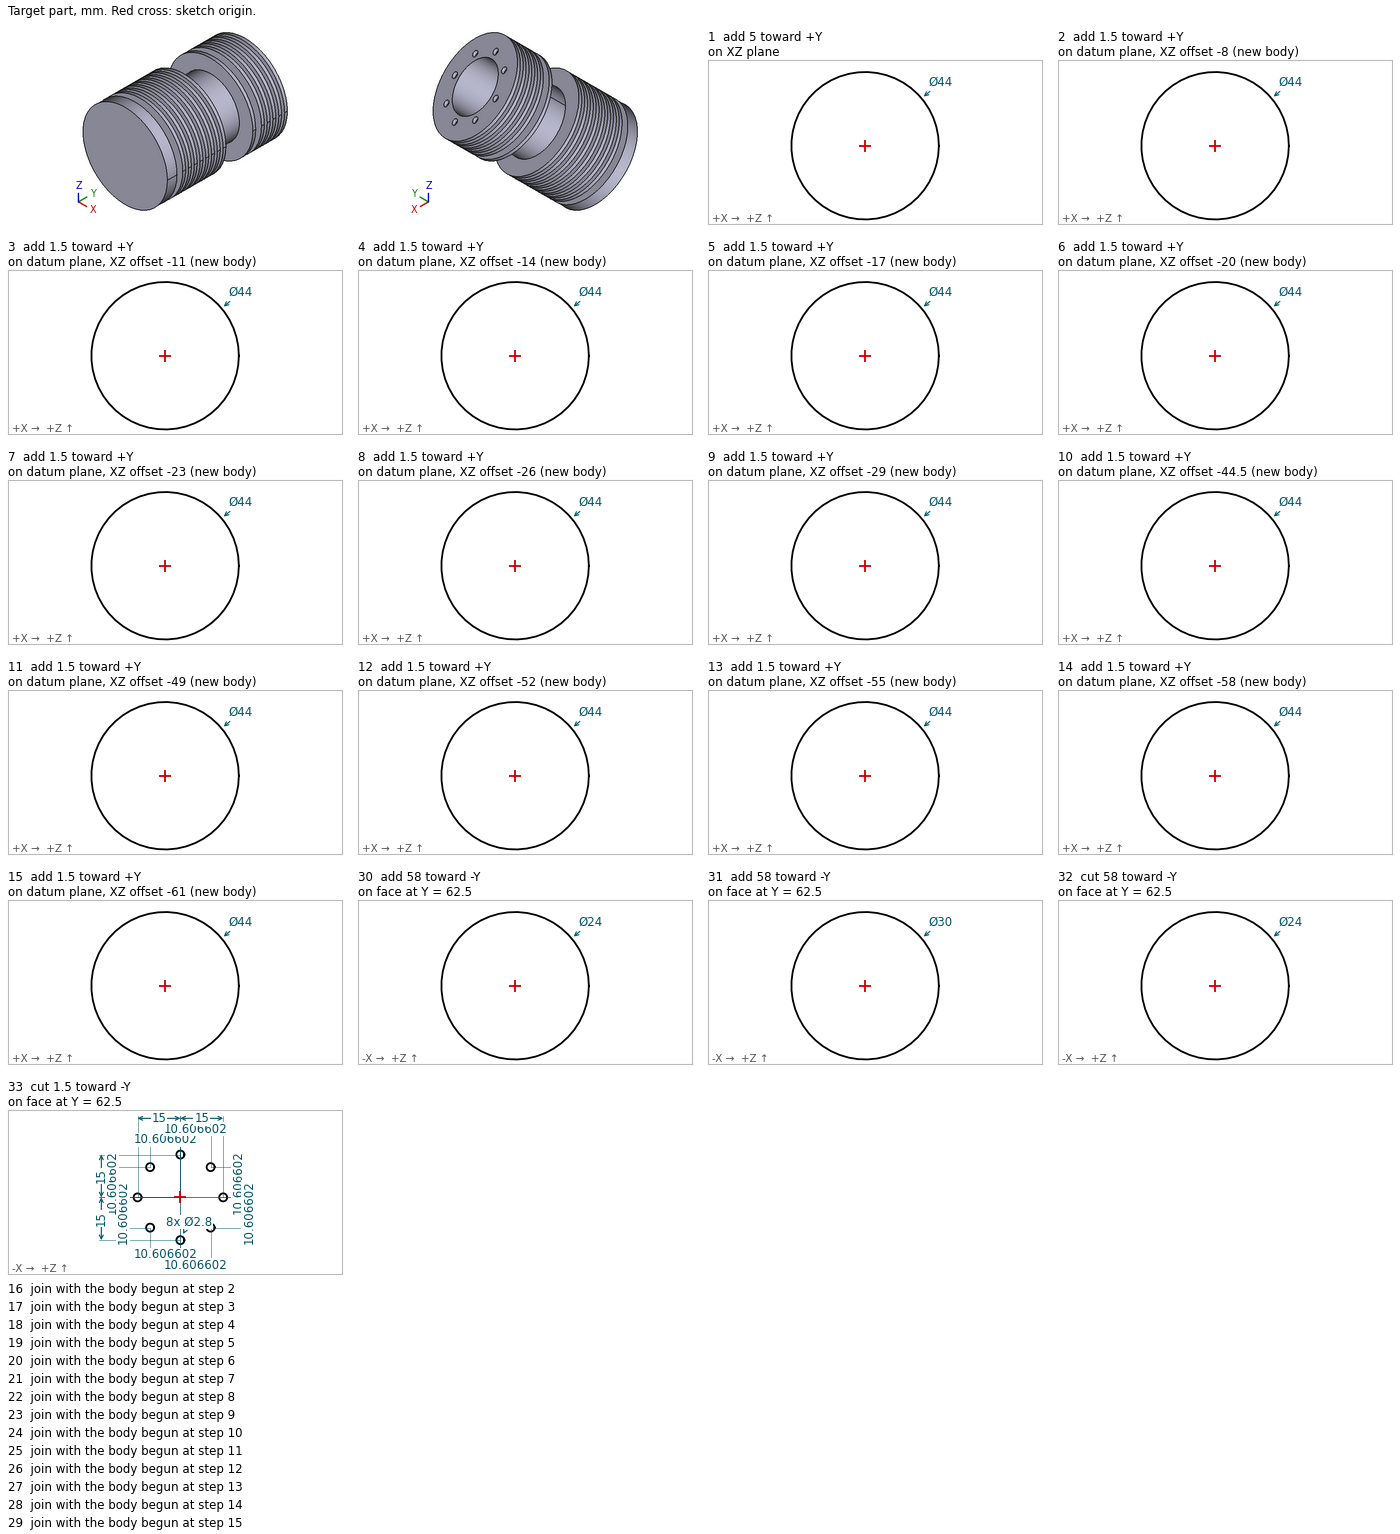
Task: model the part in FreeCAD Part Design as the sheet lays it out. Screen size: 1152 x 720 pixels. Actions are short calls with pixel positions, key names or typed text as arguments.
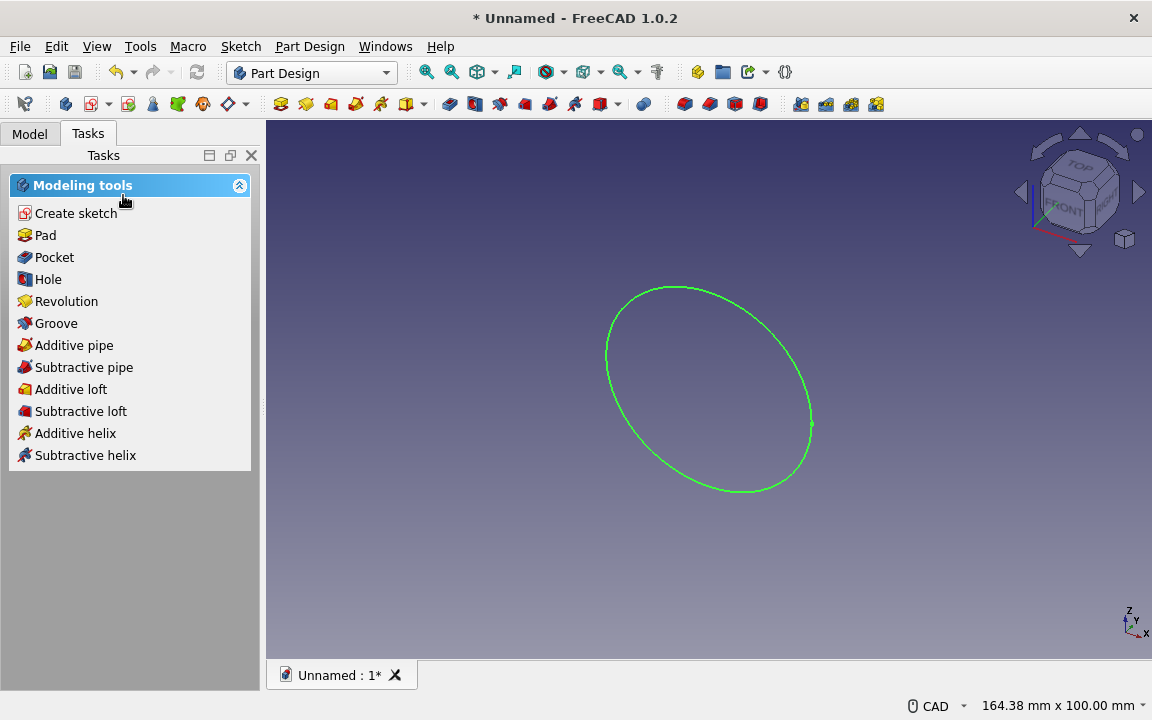
click(281, 104)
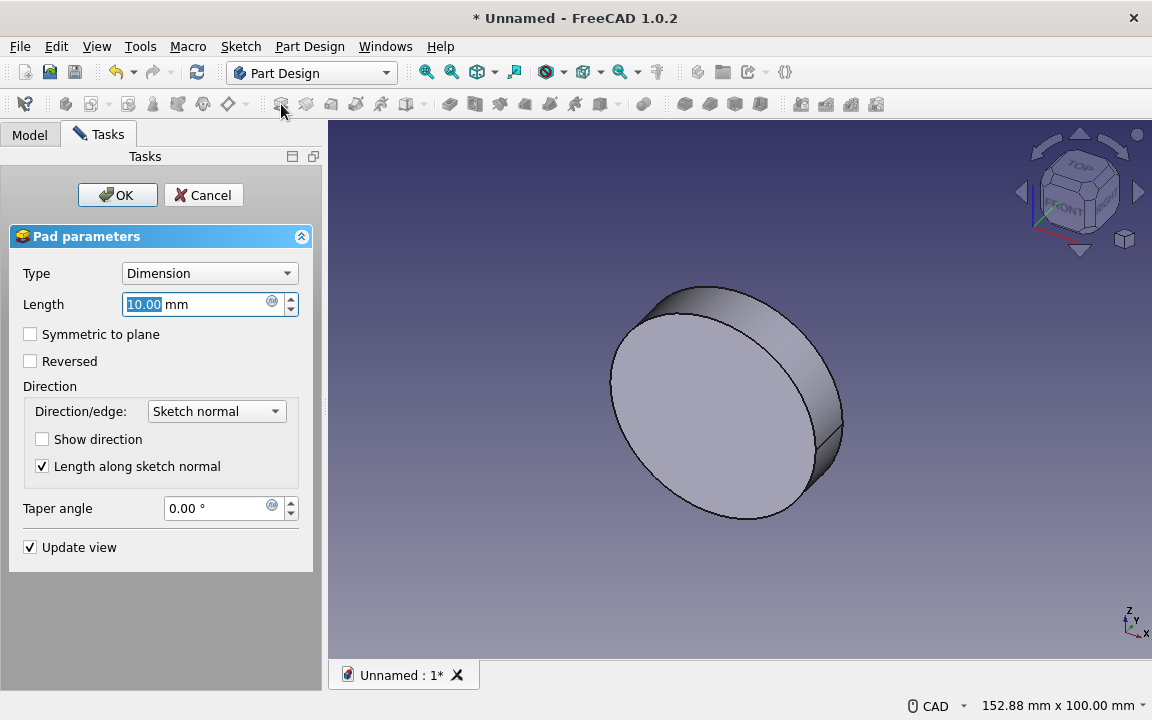
text(5)
key(Tab)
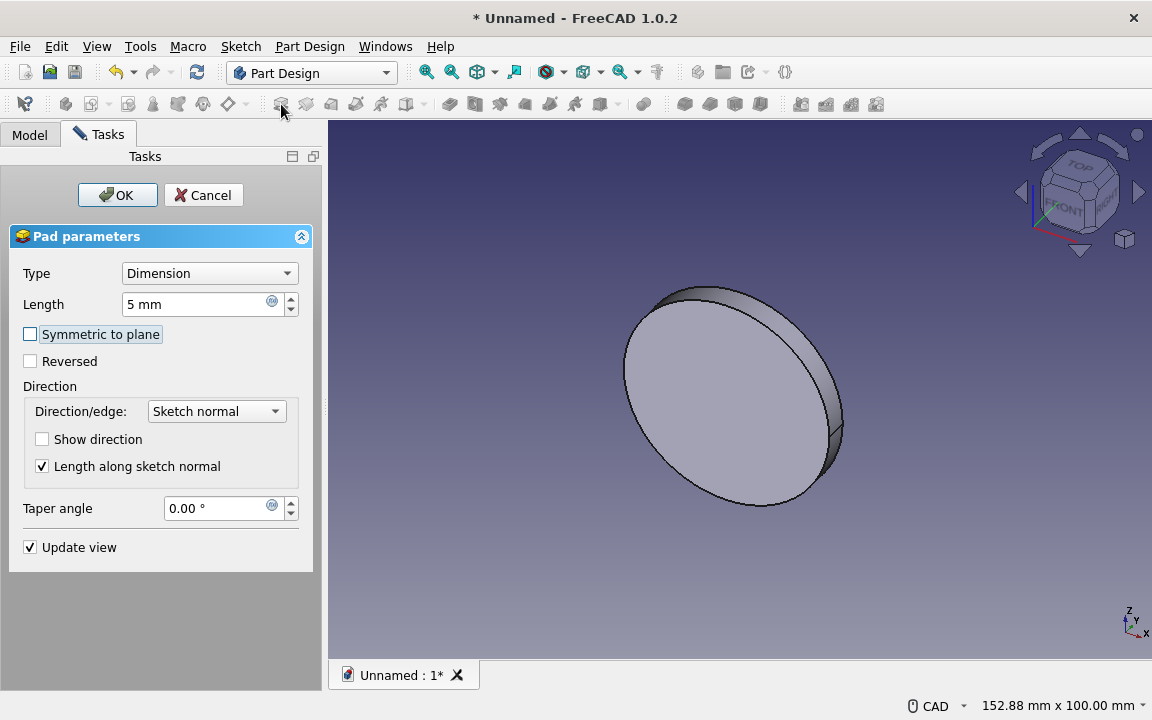
click(31, 361)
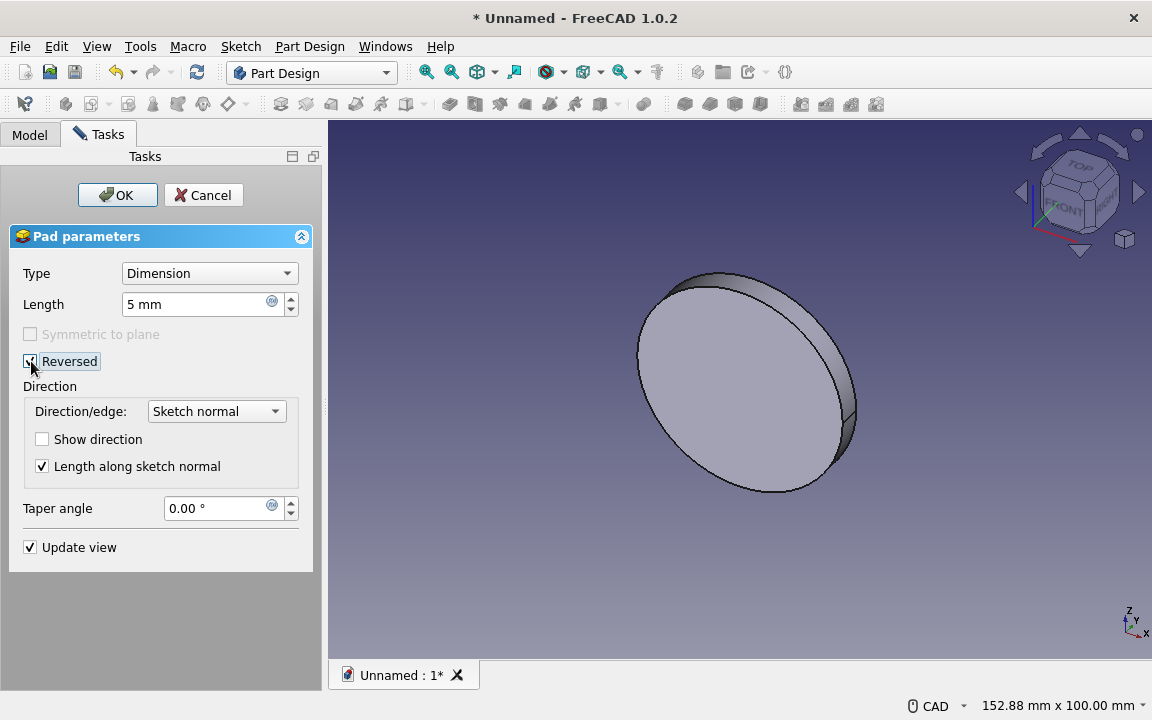
click(118, 195)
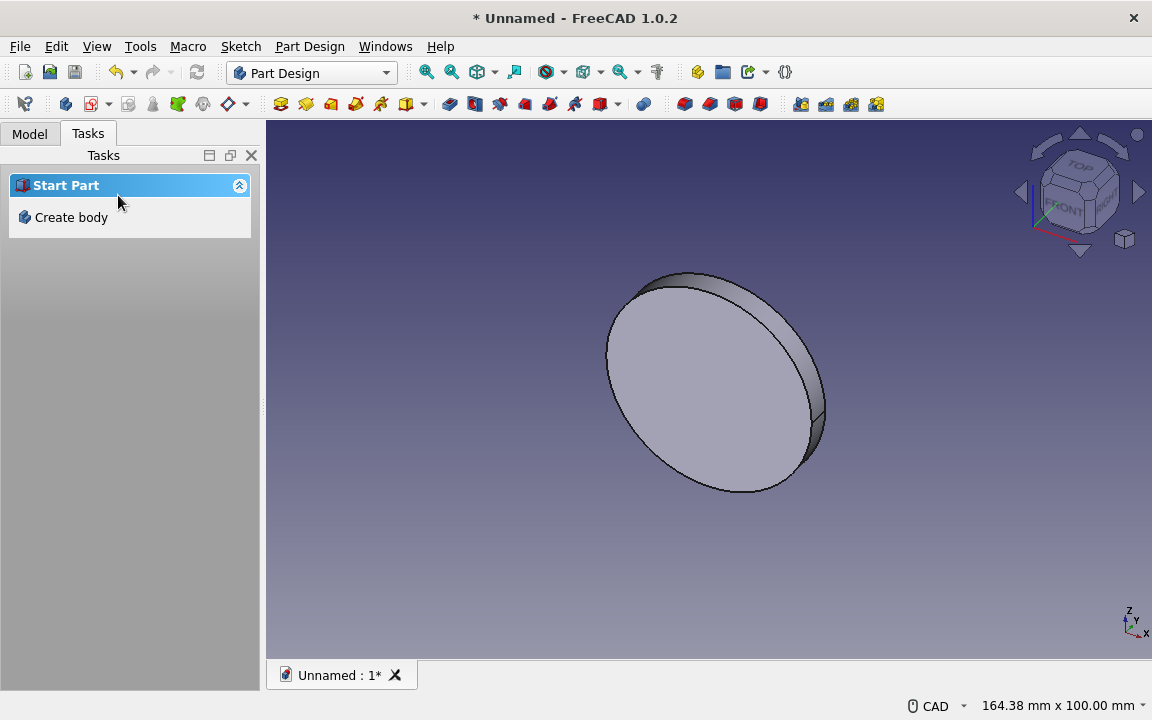
click(66, 104)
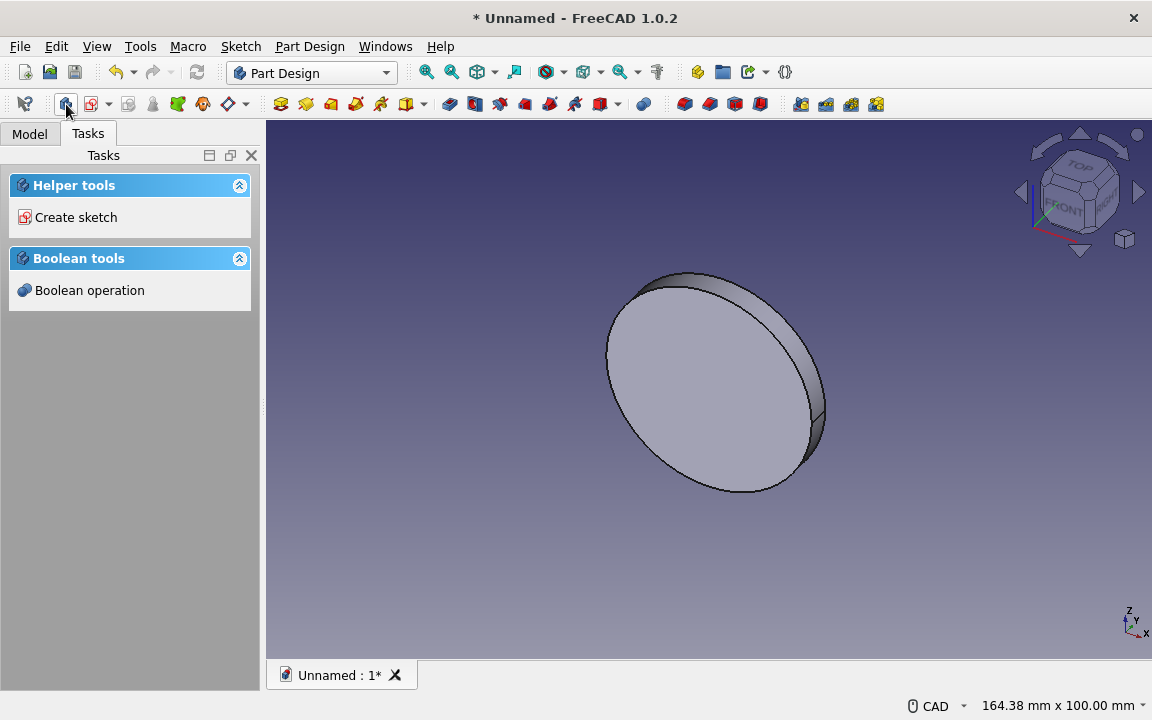
click(30, 134)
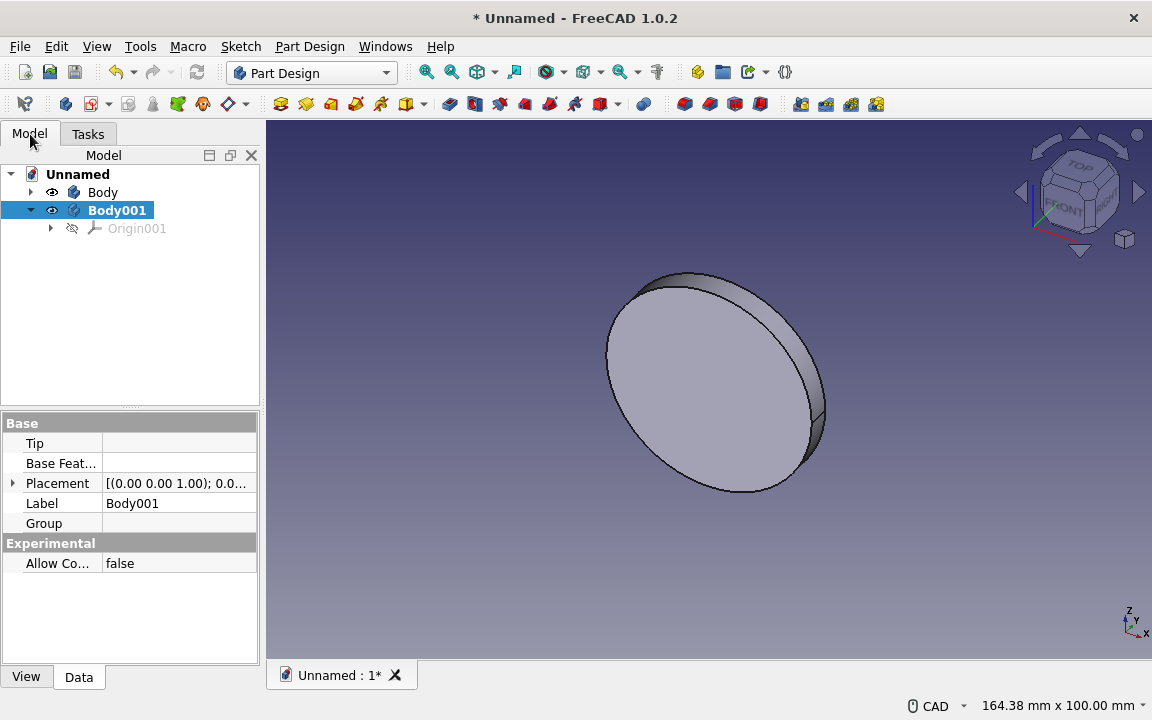
click(51, 228)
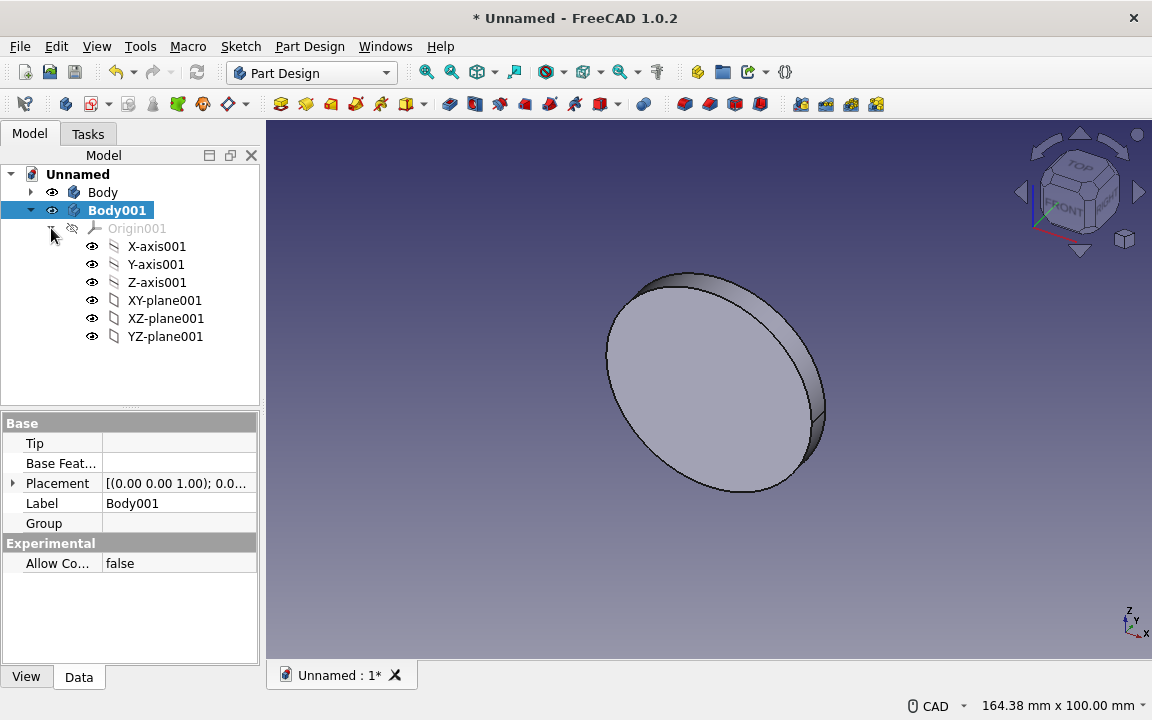
click(137, 318)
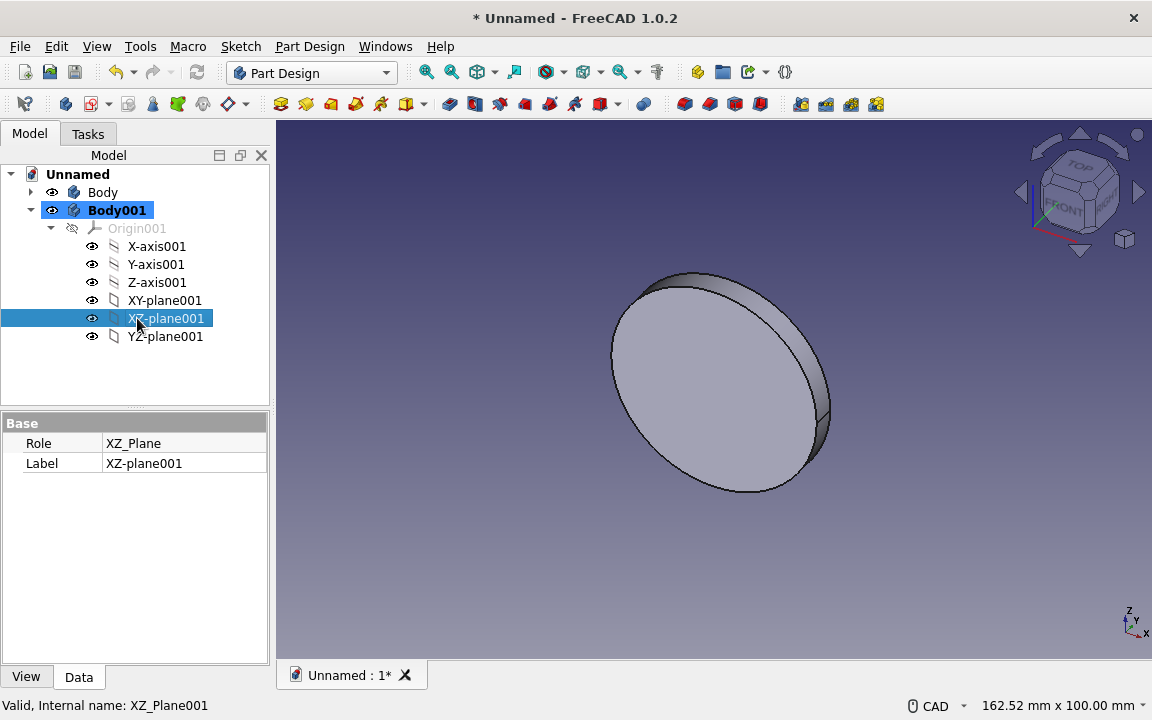
click(228, 104)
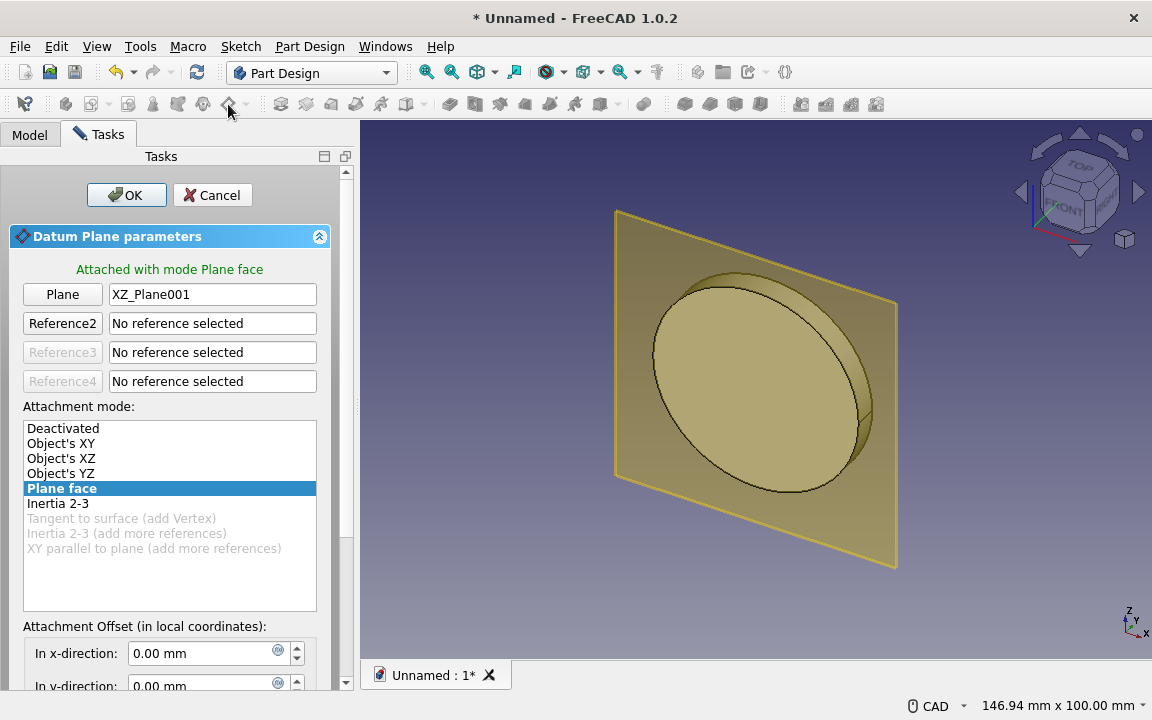
scroll(346, 428, down, 2)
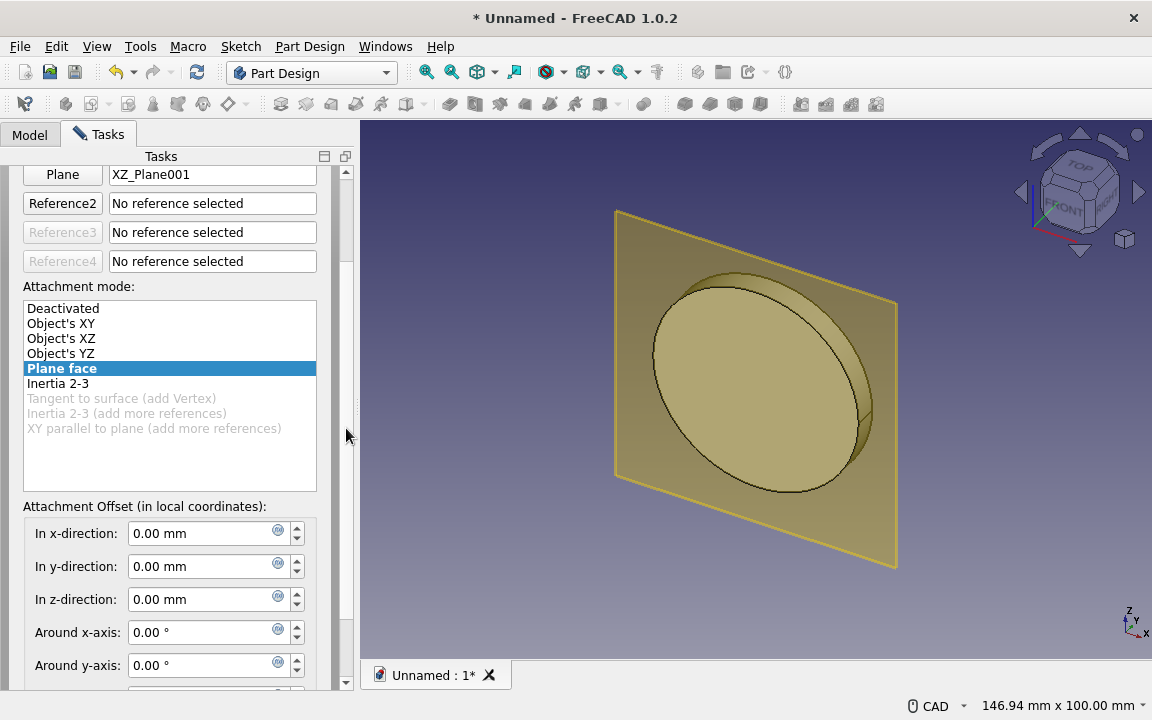
triple_click(210, 600)